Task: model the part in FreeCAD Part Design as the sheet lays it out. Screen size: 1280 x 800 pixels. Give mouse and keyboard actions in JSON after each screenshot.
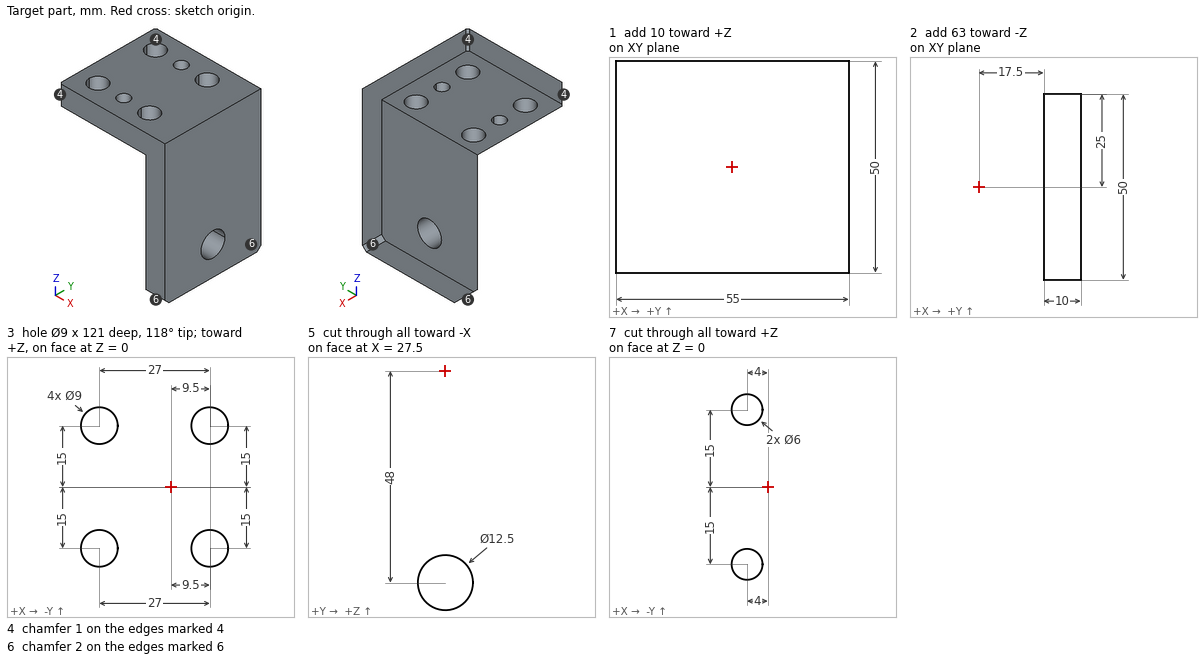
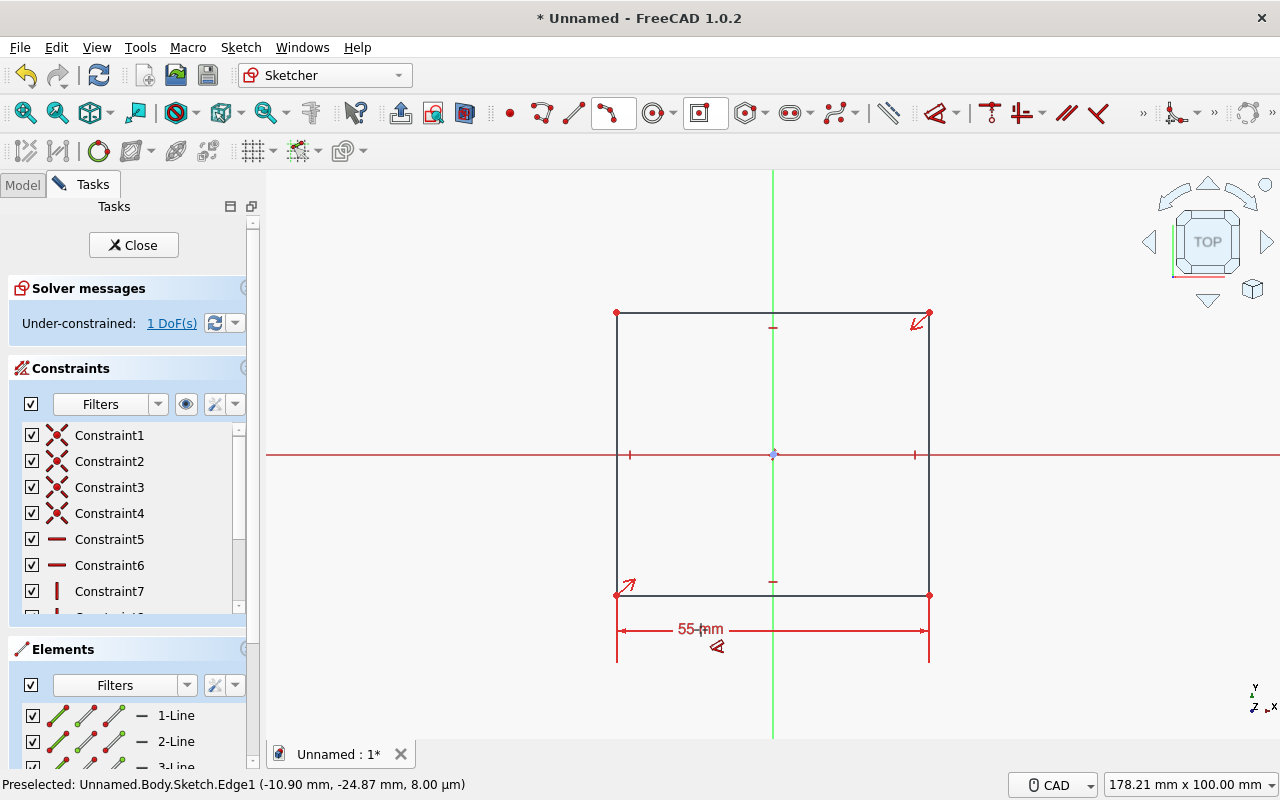
{"action": "left_click", "coordinate": [929, 511]}
{"action": "left_click", "coordinate": [963, 389]}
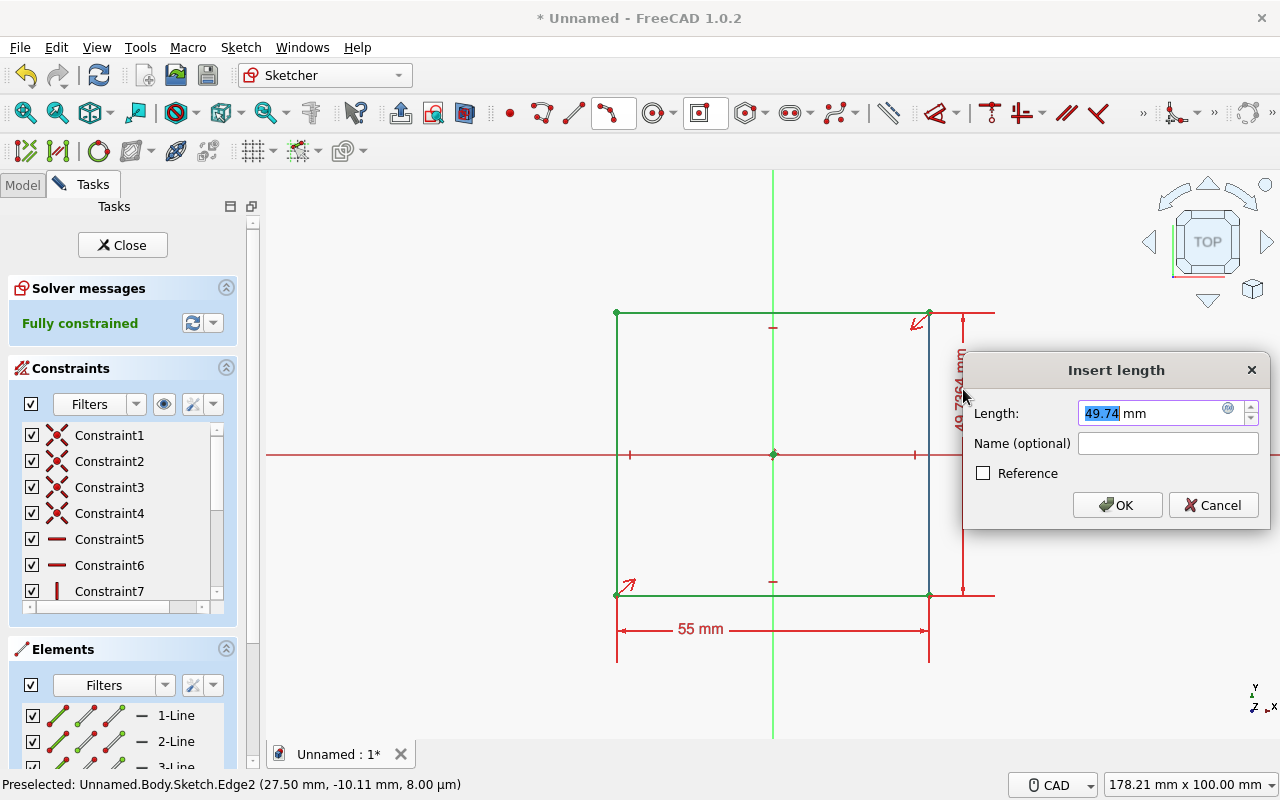
{"action": "type", "text": "50"}
{"action": "key", "text": "Return"}
{"action": "key", "text": "Escape"}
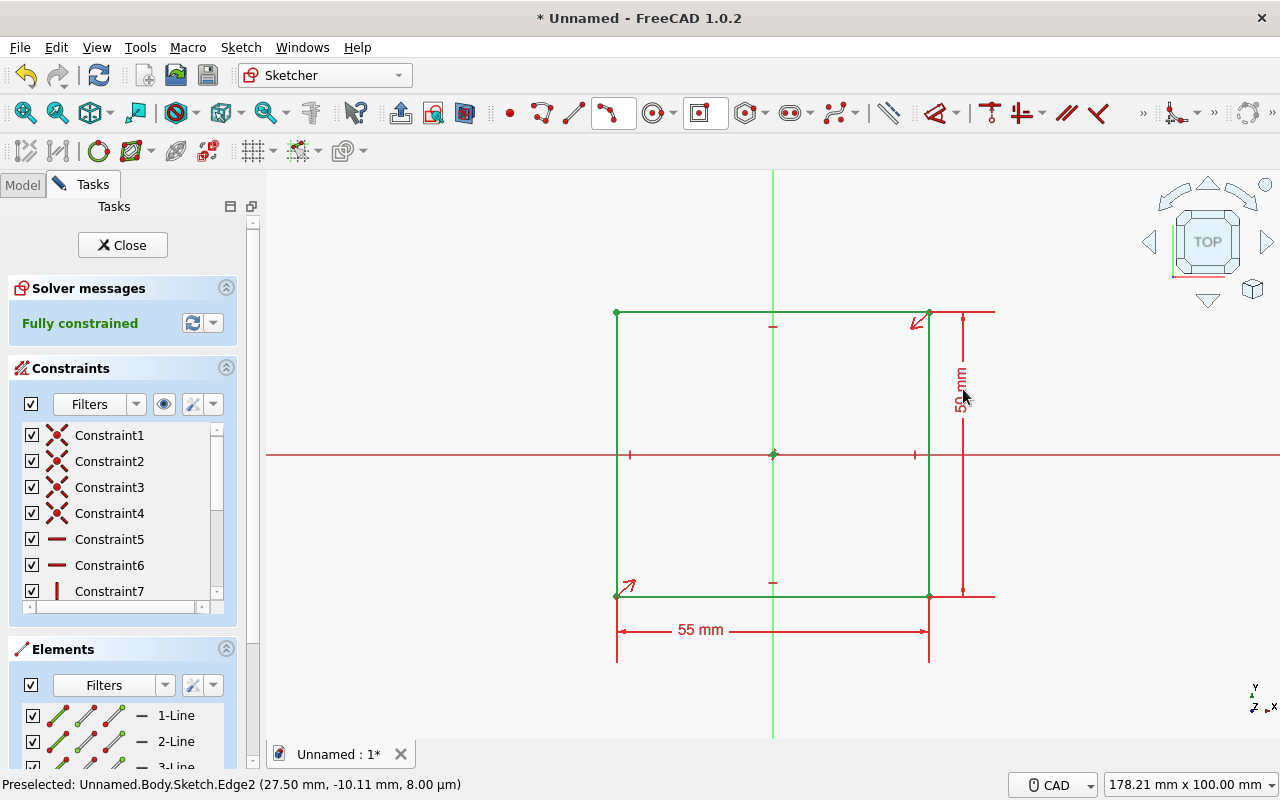
{"action": "left_click", "coordinate": [123, 245]}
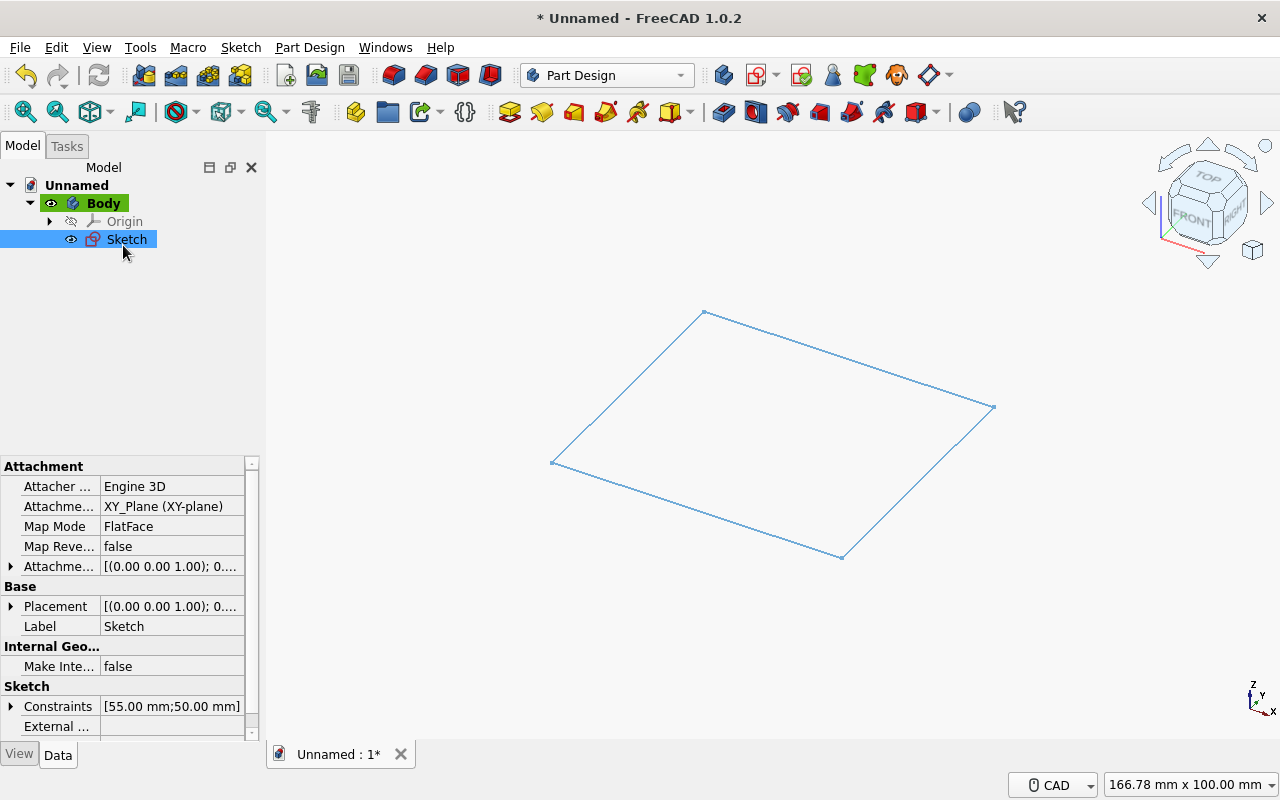
{"action": "left_click", "coordinate": [510, 112]}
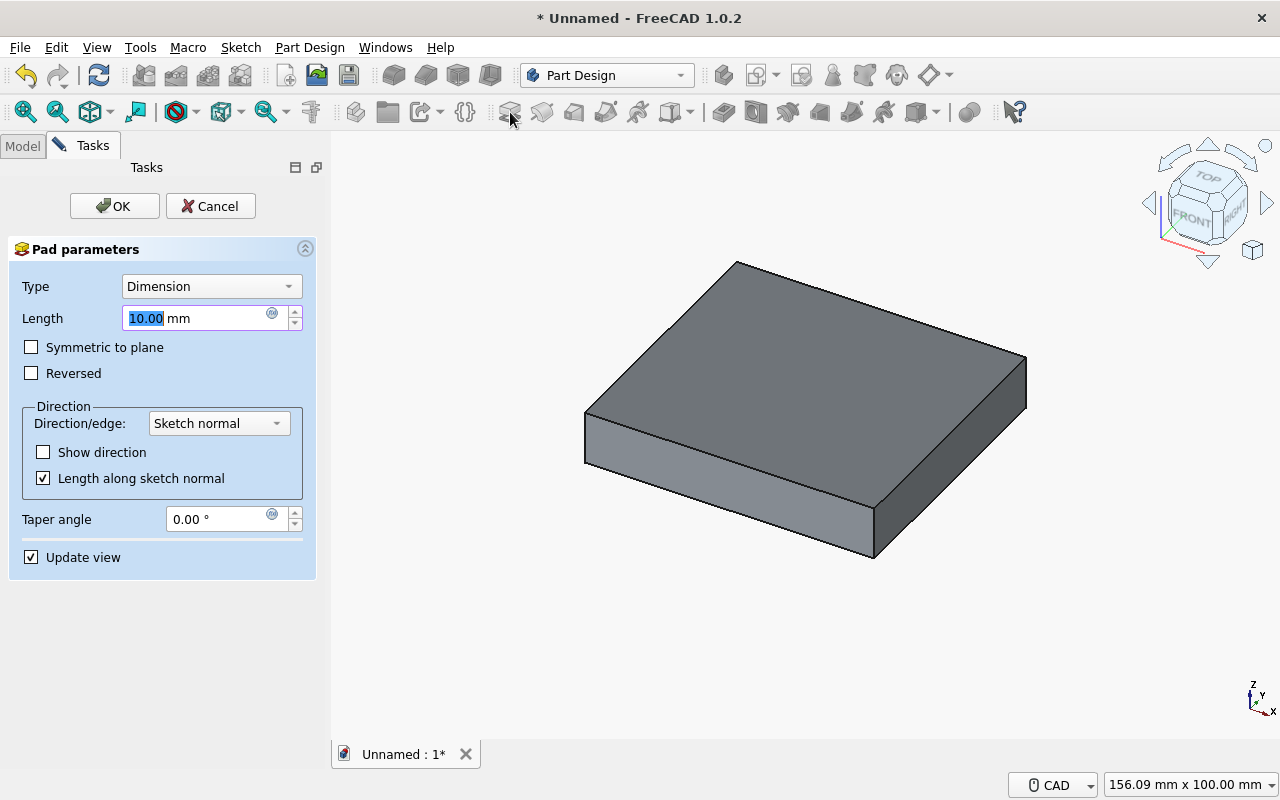
{"action": "type", "text": "10"}
{"action": "key", "text": "Tab"}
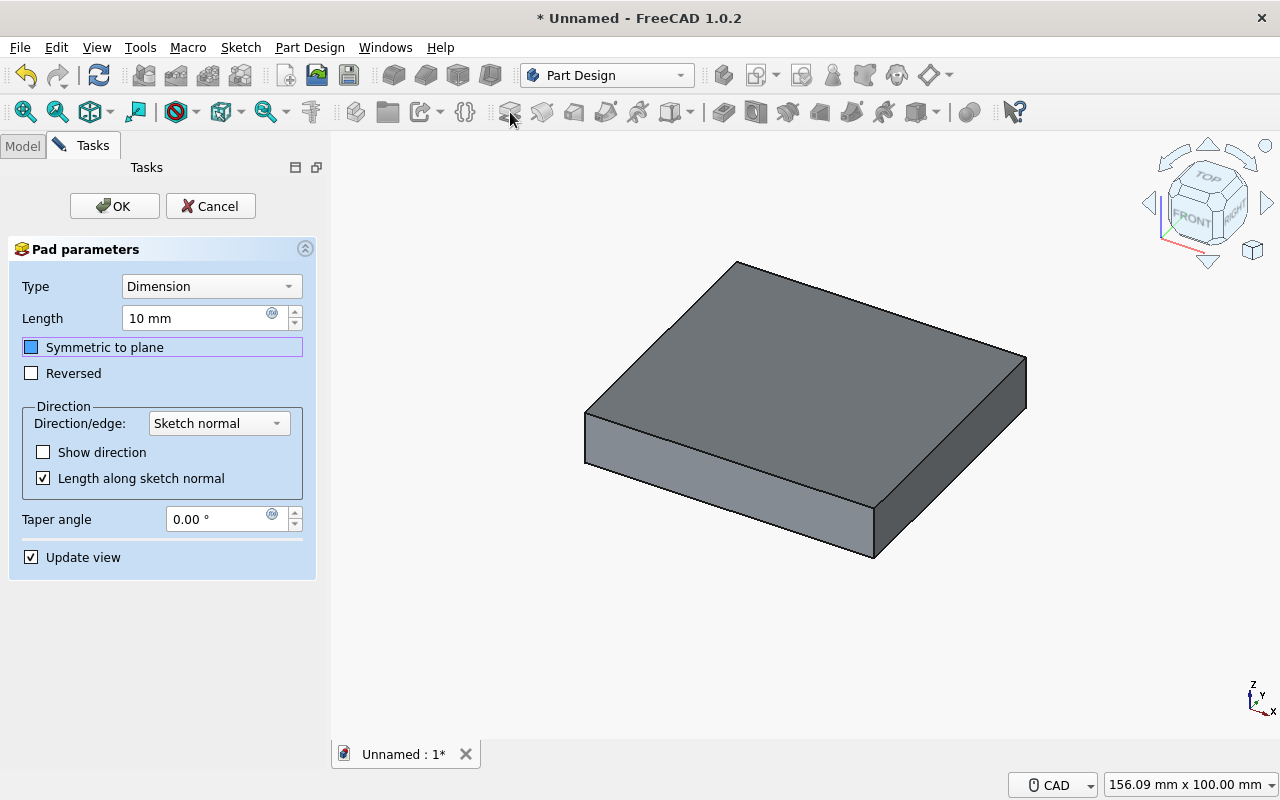
{"action": "left_click", "coordinate": [115, 206]}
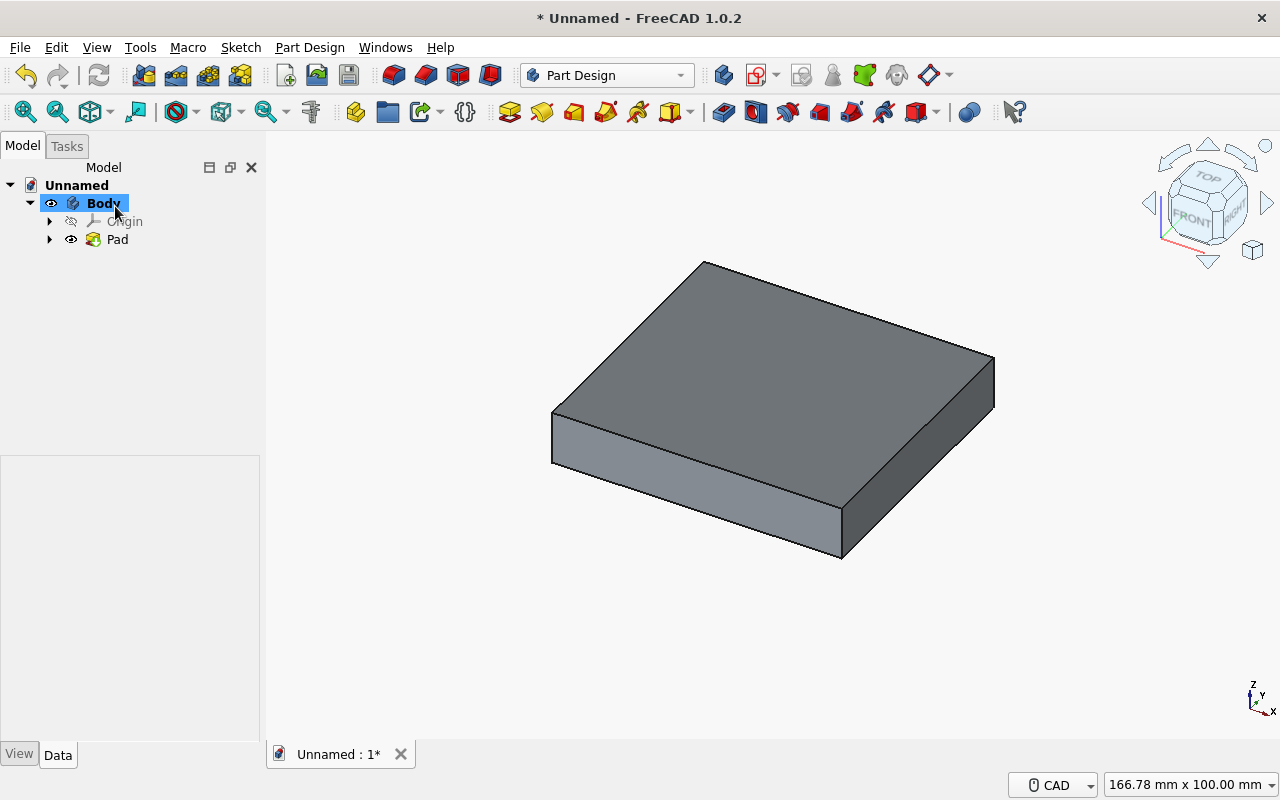
{"action": "left_click", "coordinate": [756, 76]}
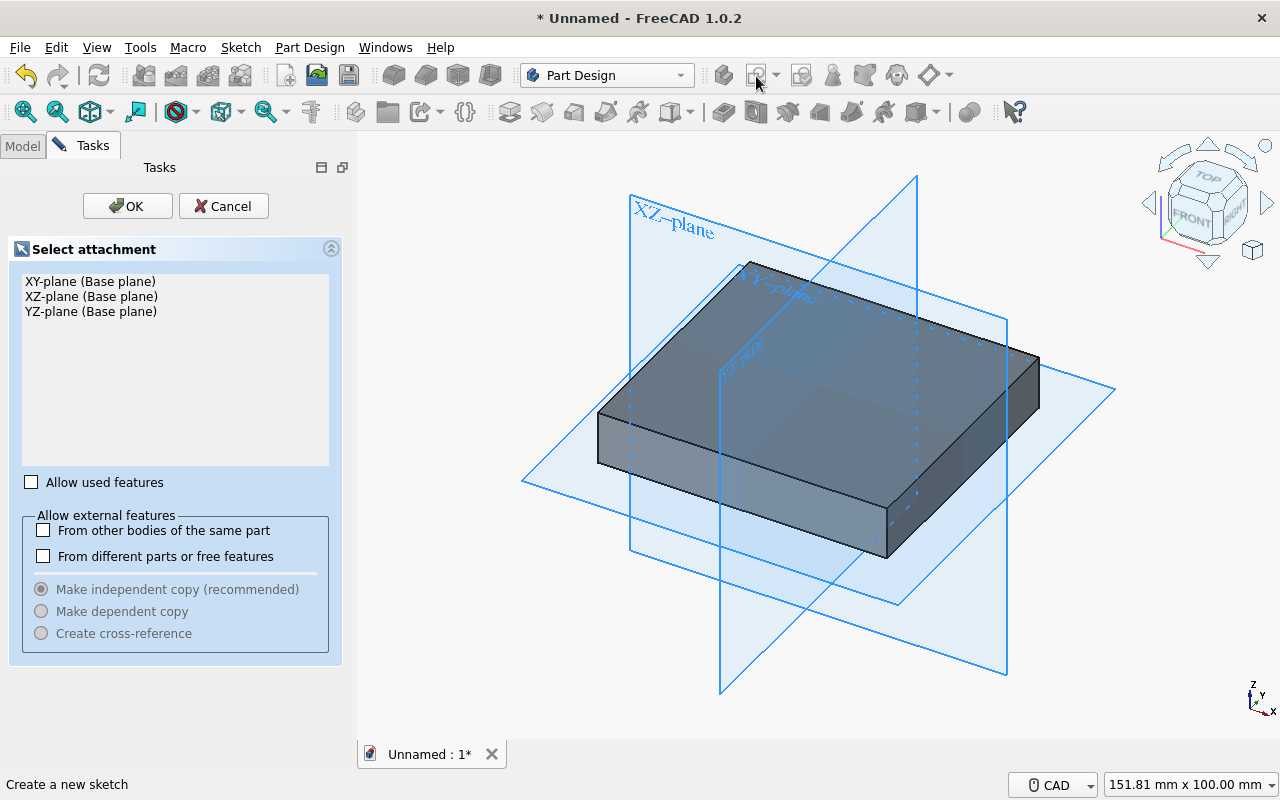
{"action": "left_click", "coordinate": [82, 282]}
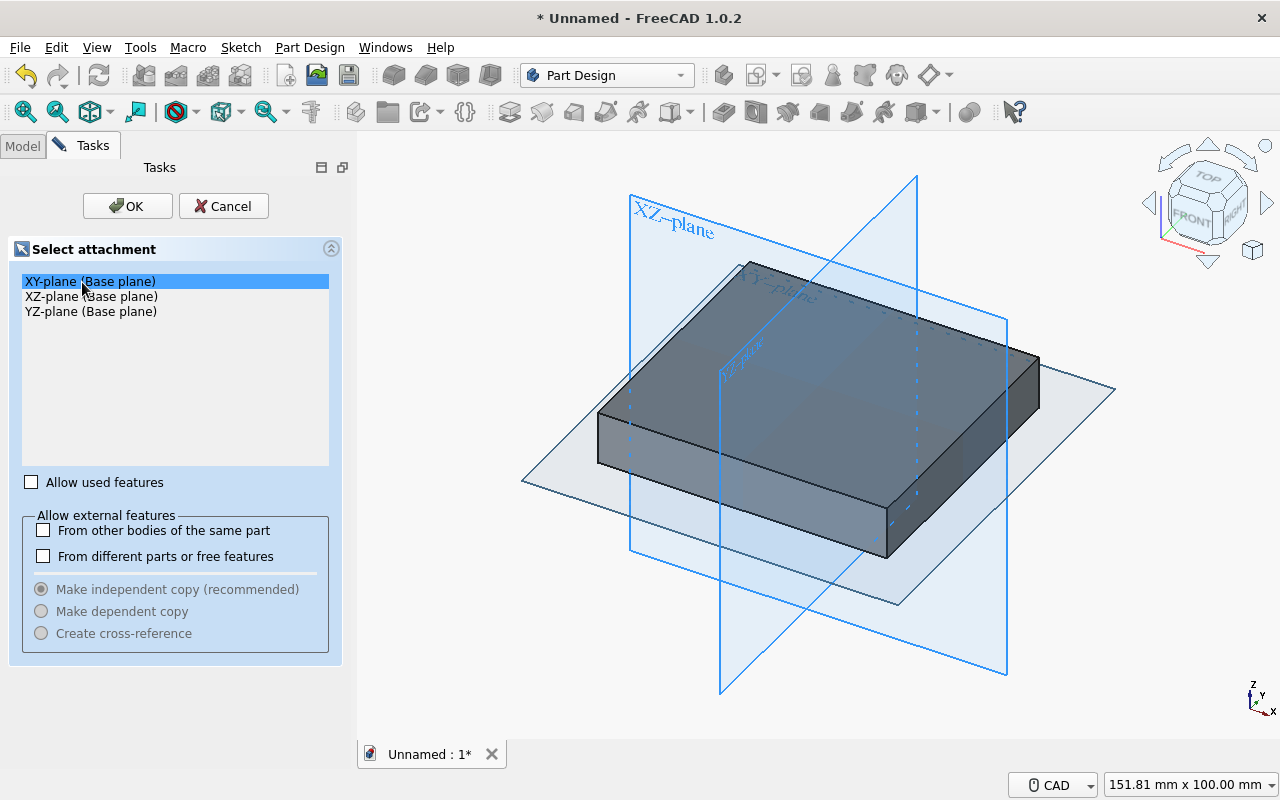
{"action": "left_click", "coordinate": [128, 206]}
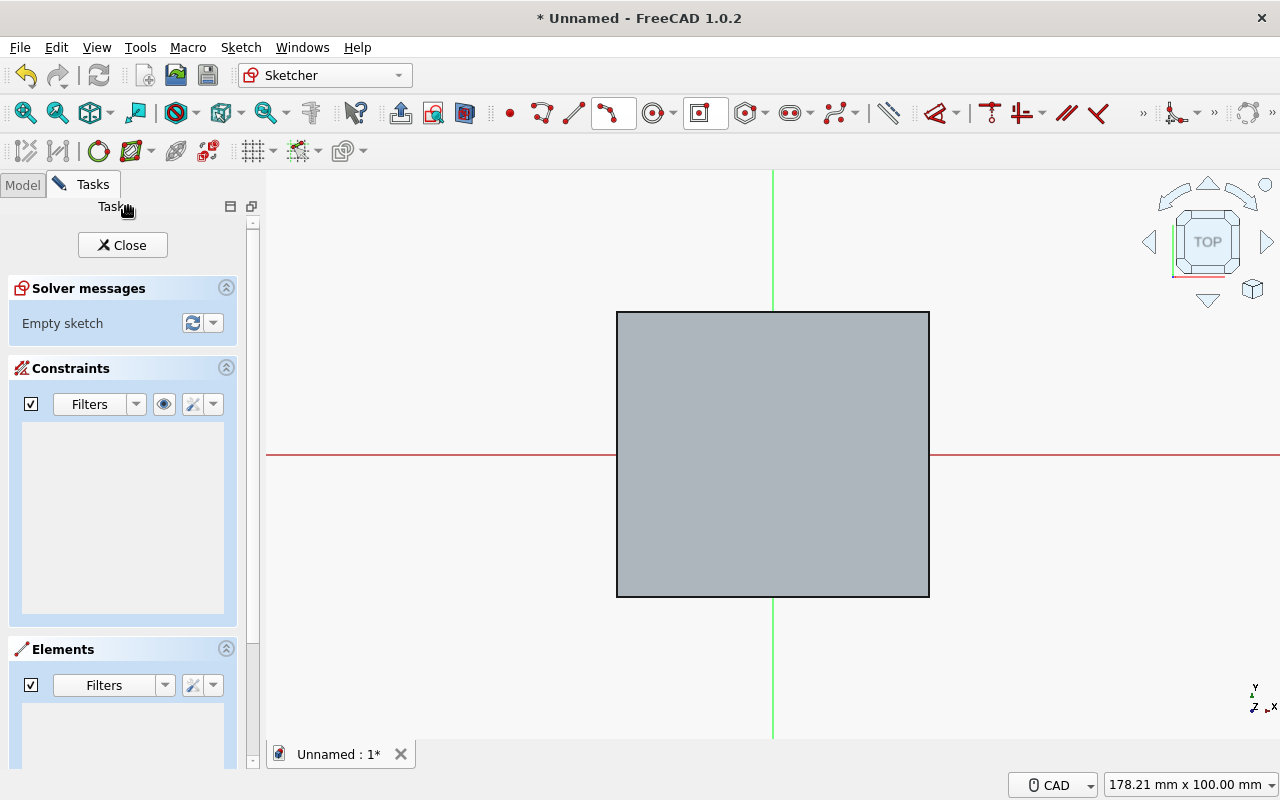
{"action": "left_click", "coordinate": [466, 114]}